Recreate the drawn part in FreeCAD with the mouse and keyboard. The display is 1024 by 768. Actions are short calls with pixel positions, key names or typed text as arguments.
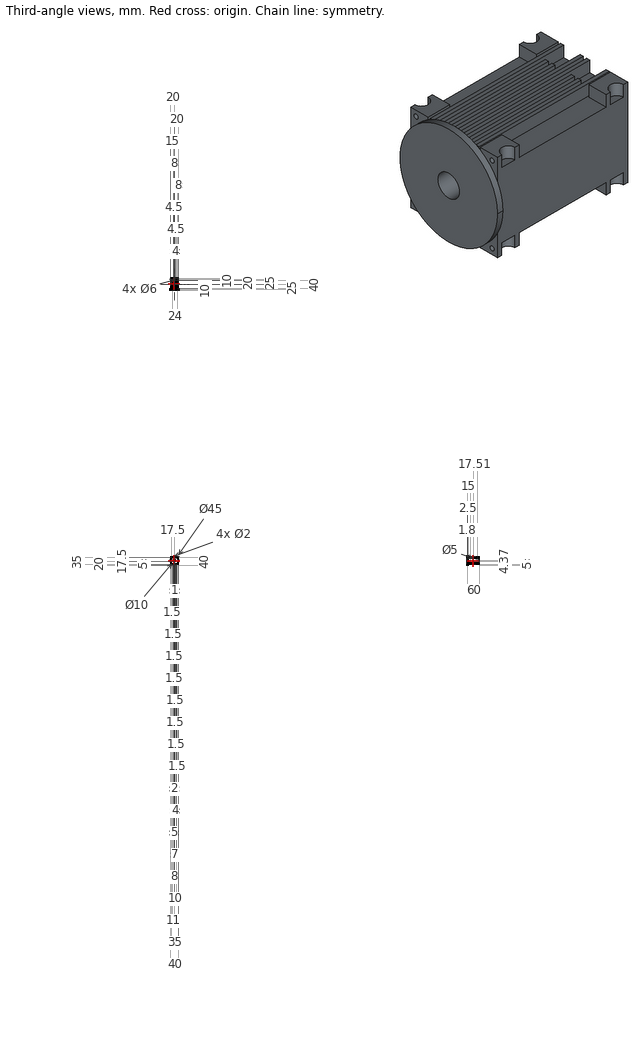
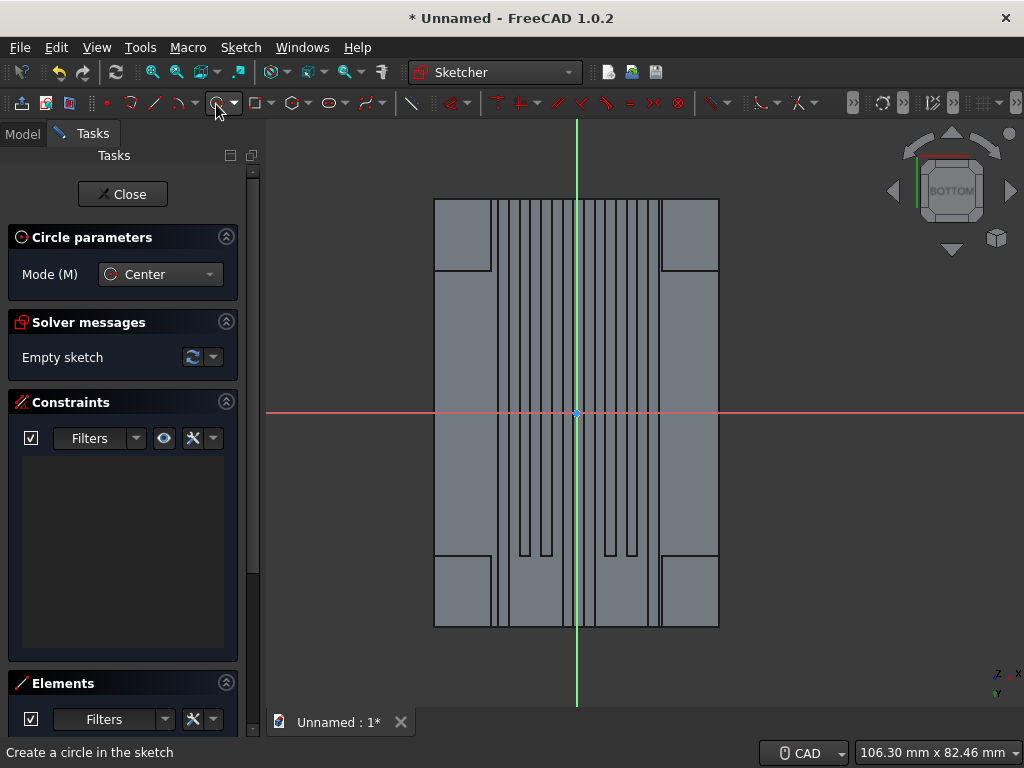
click(719, 592)
click(735, 577)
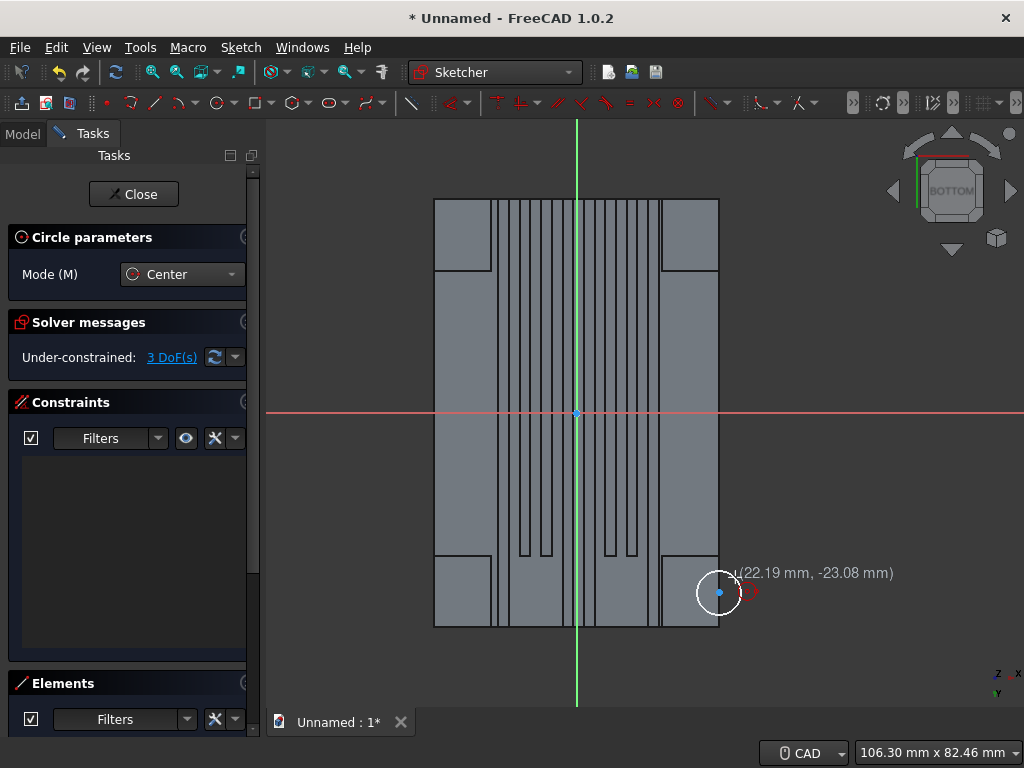
click(434, 592)
click(449, 577)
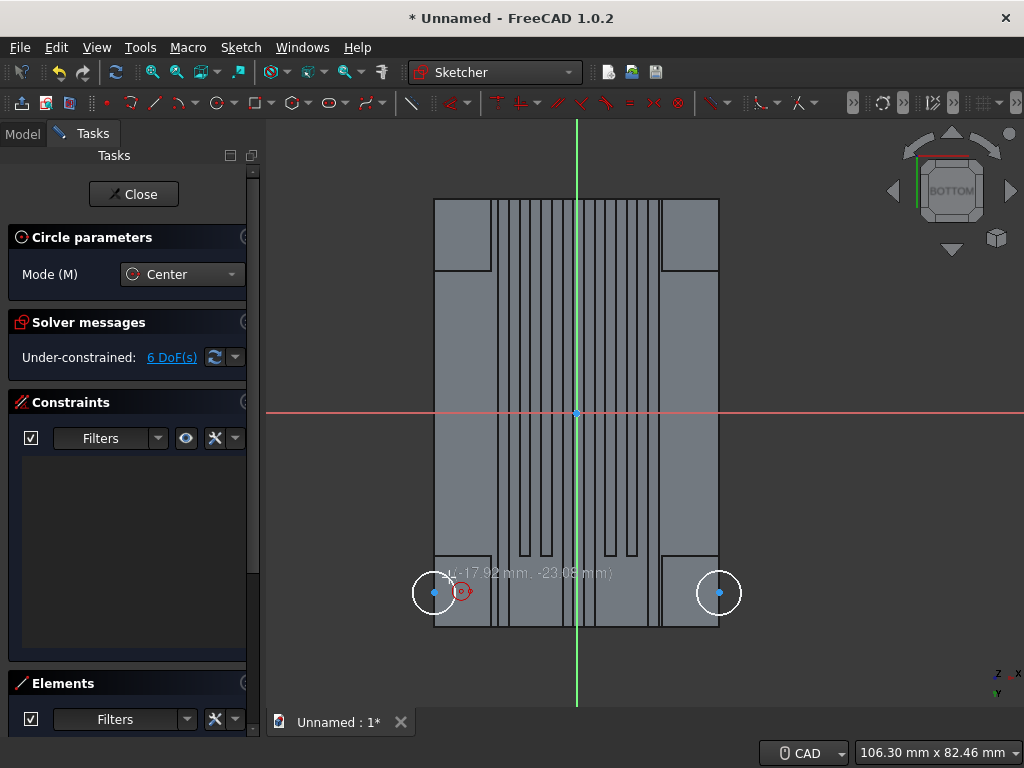
click(719, 235)
click(735, 220)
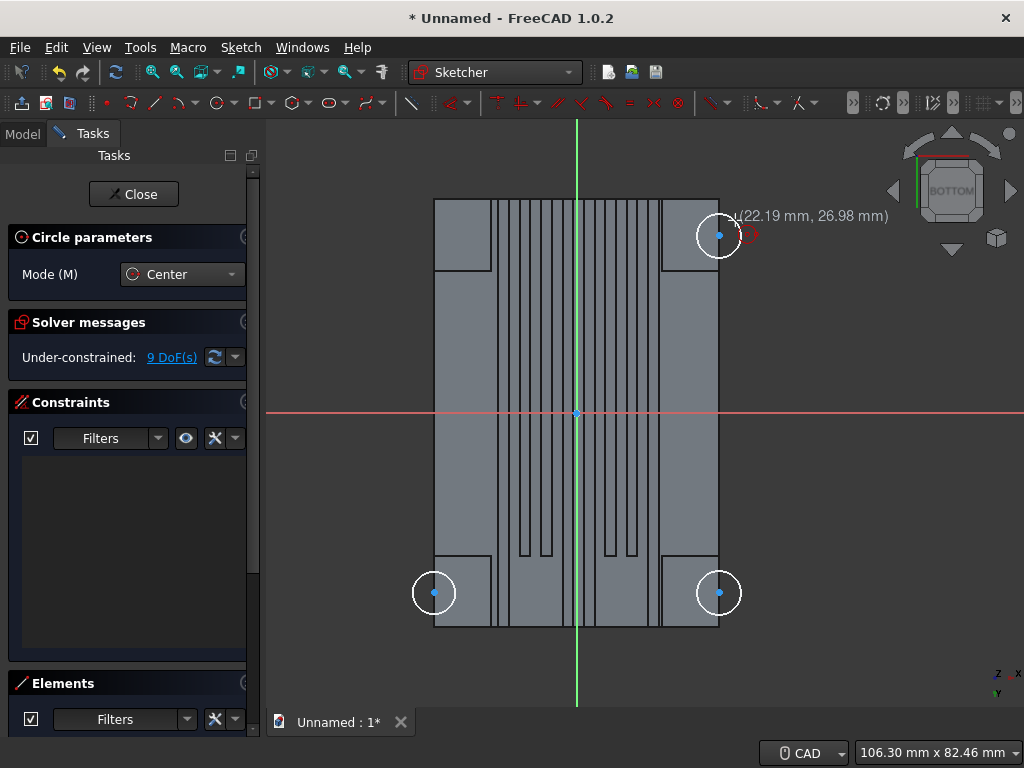
click(434, 235)
click(449, 220)
key(Escape)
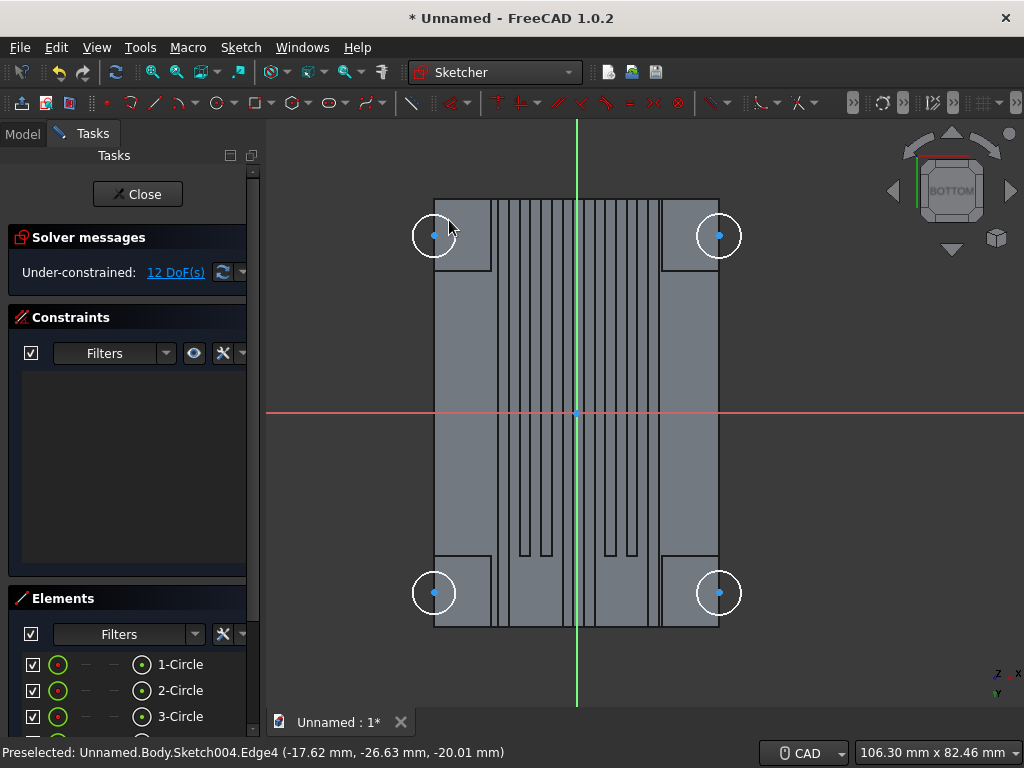
click(734, 577)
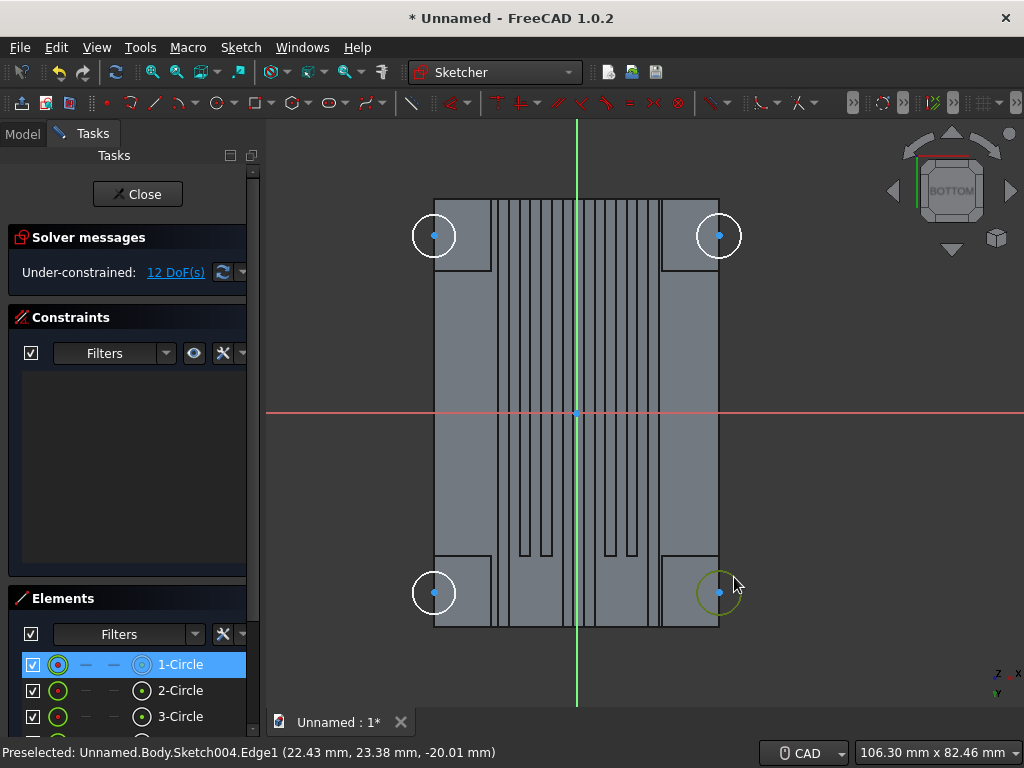
click(449, 578)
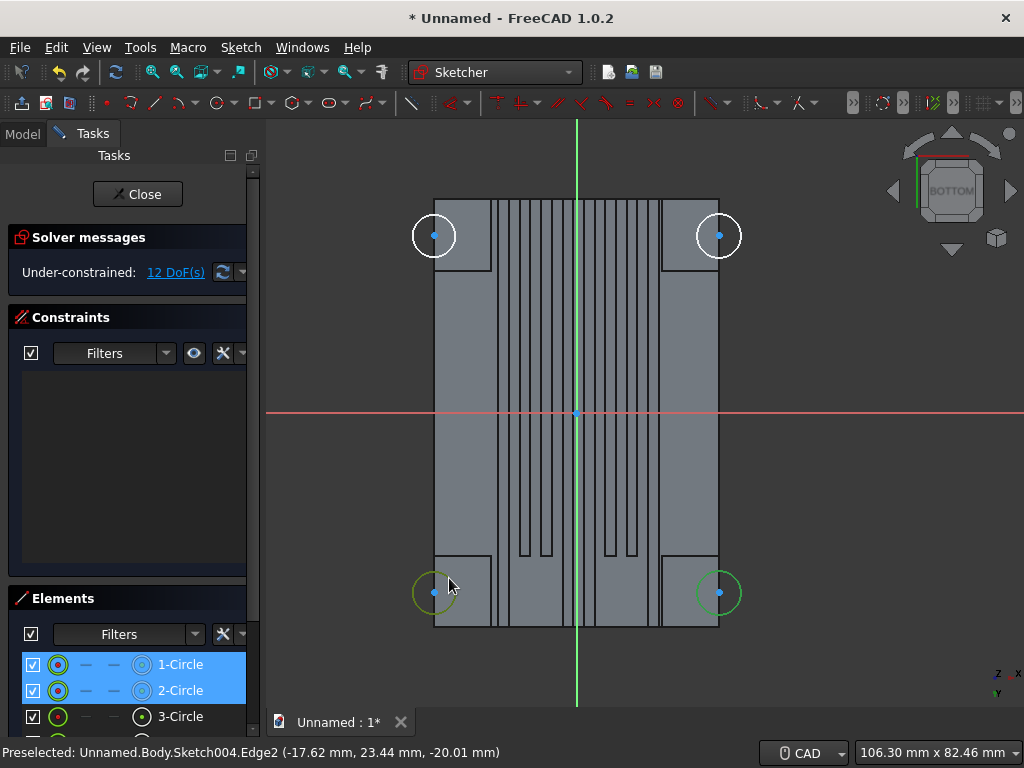
click(734, 220)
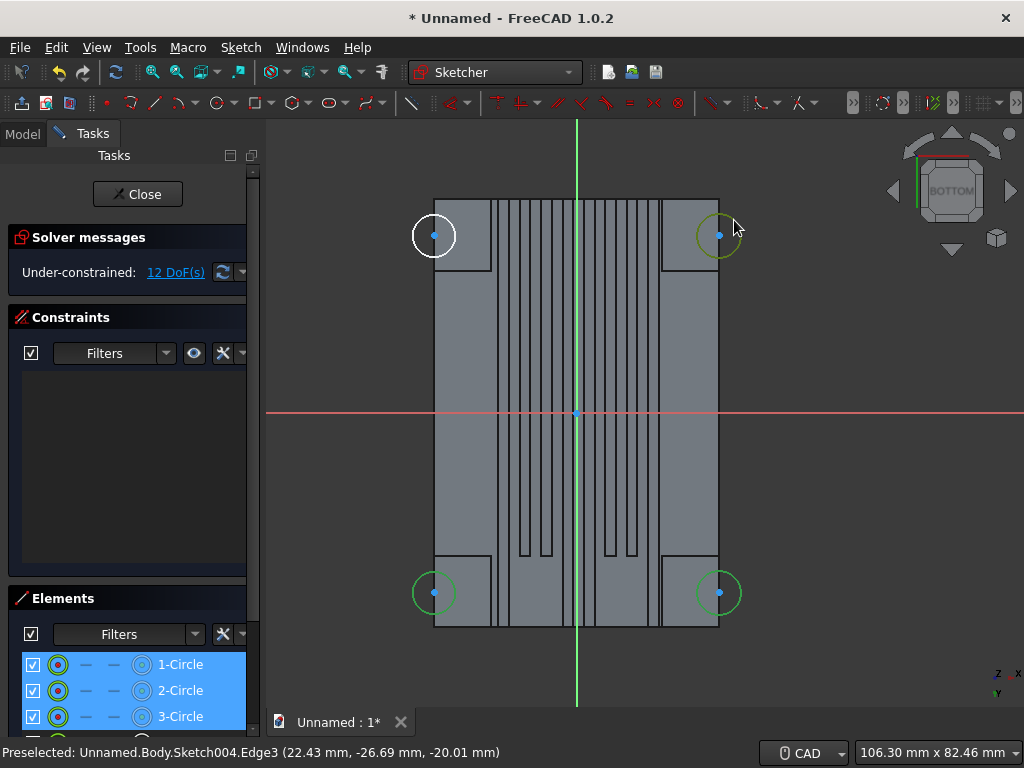
click(449, 221)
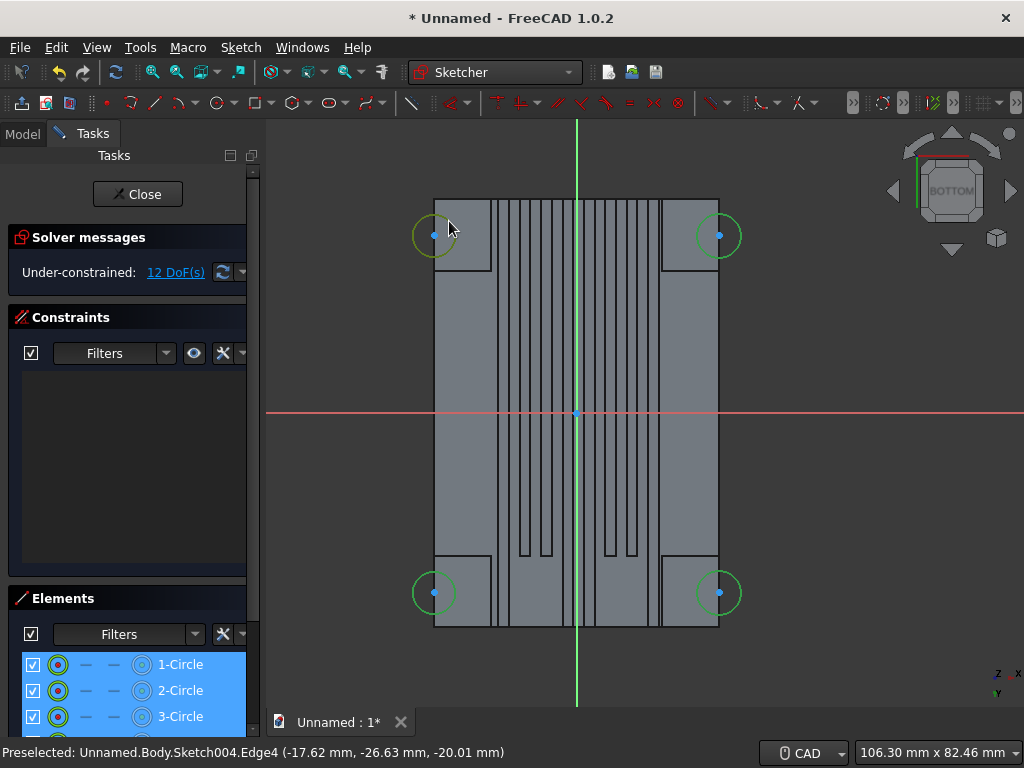
click(630, 104)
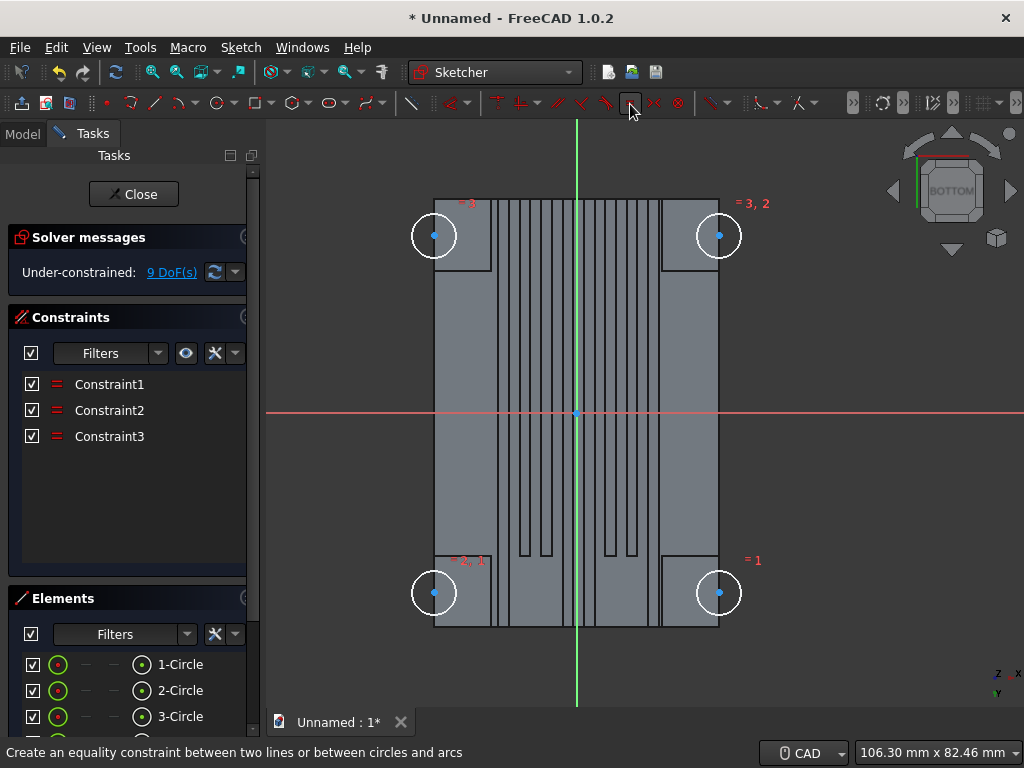
click(719, 593)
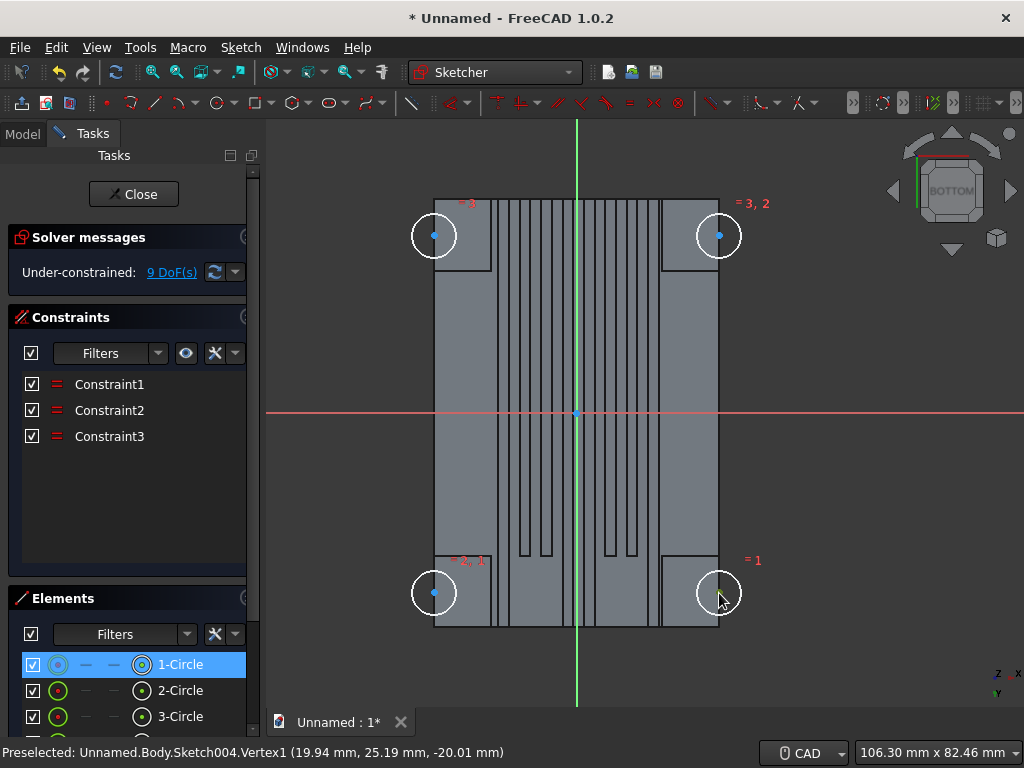
click(434, 593)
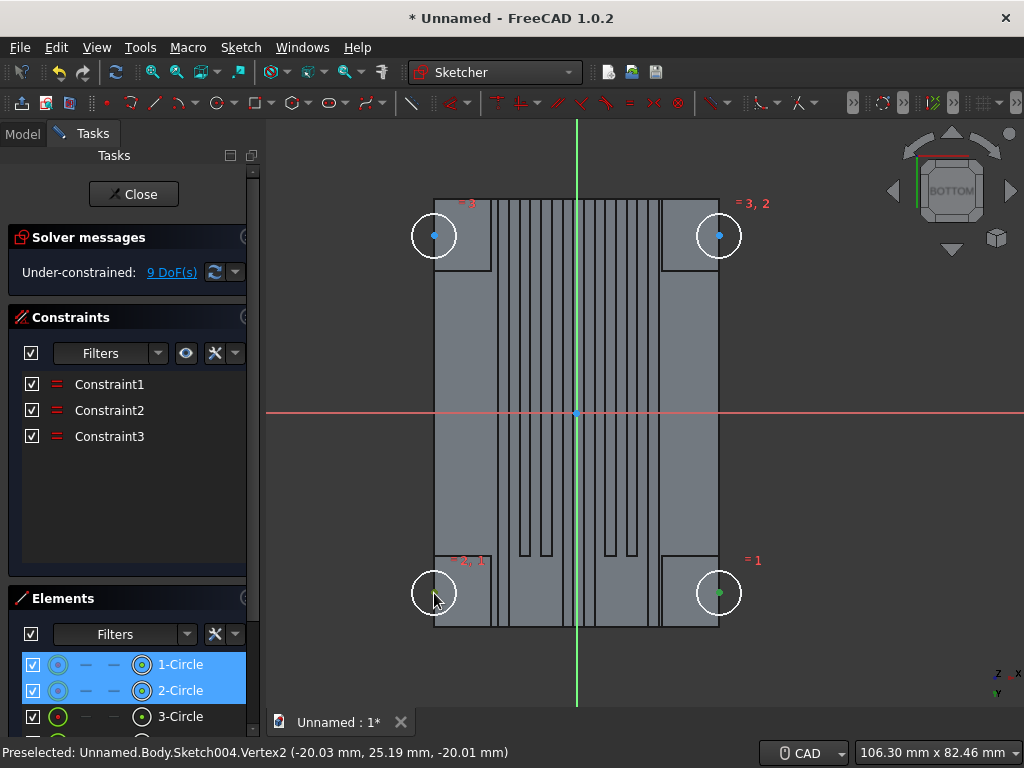
key(h)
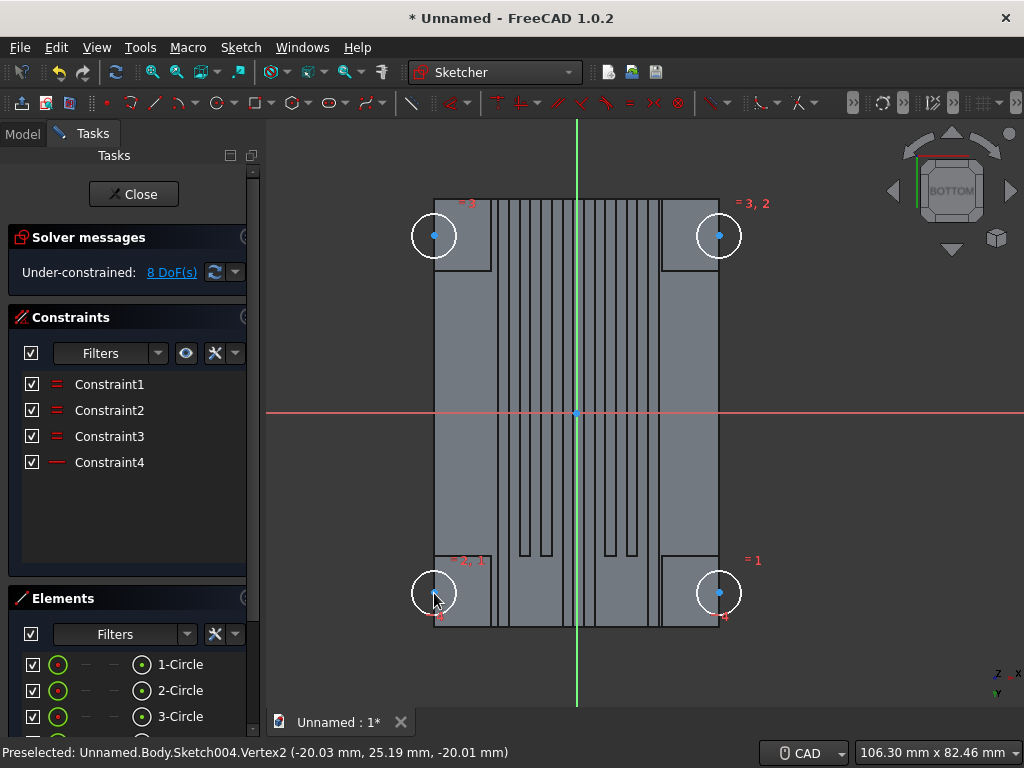
click(719, 593)